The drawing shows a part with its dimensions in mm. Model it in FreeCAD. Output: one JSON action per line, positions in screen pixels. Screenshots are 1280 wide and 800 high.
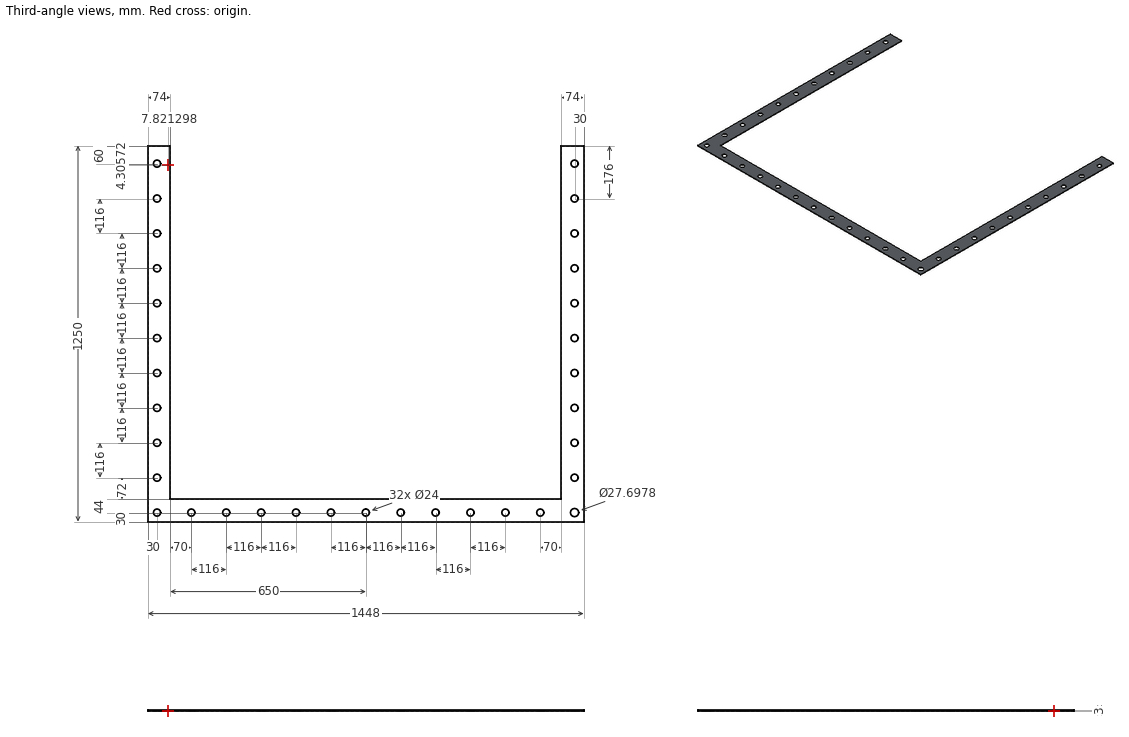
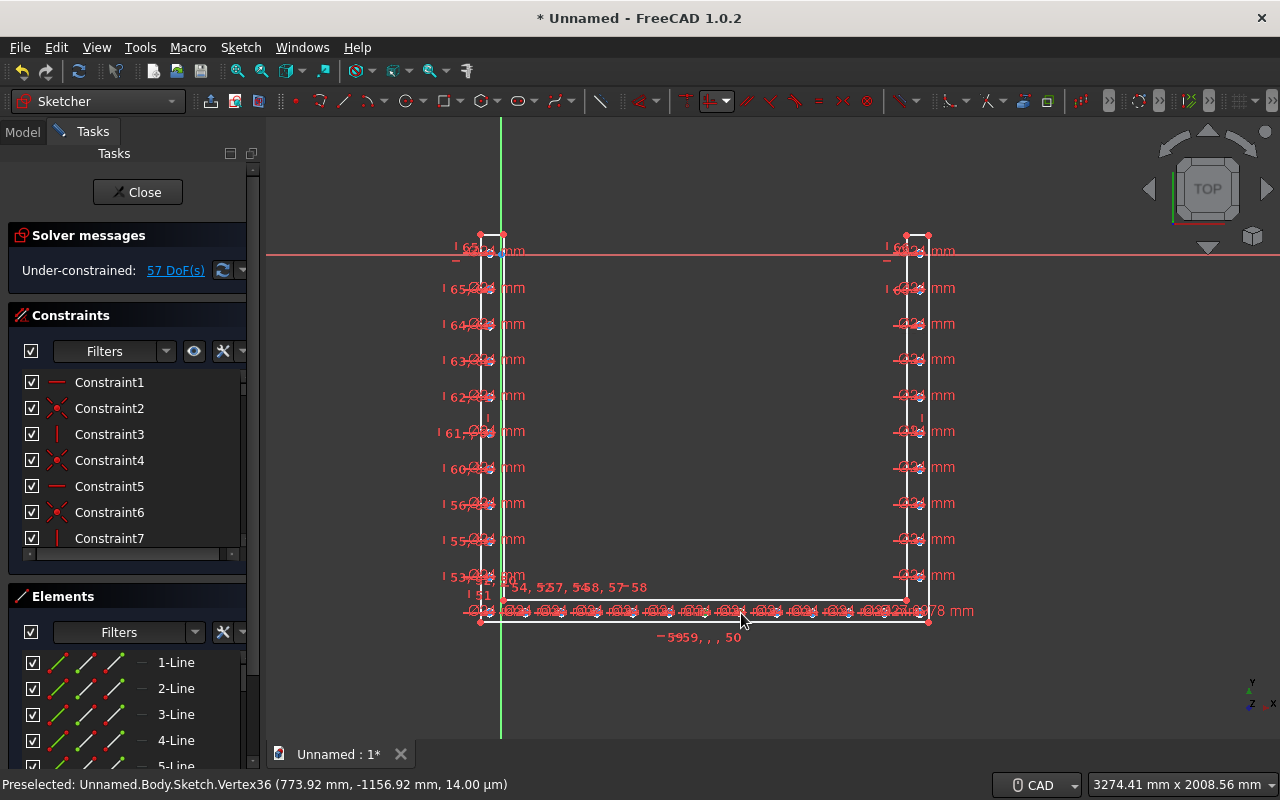
{"action": "left_click", "coordinate": [728, 102]}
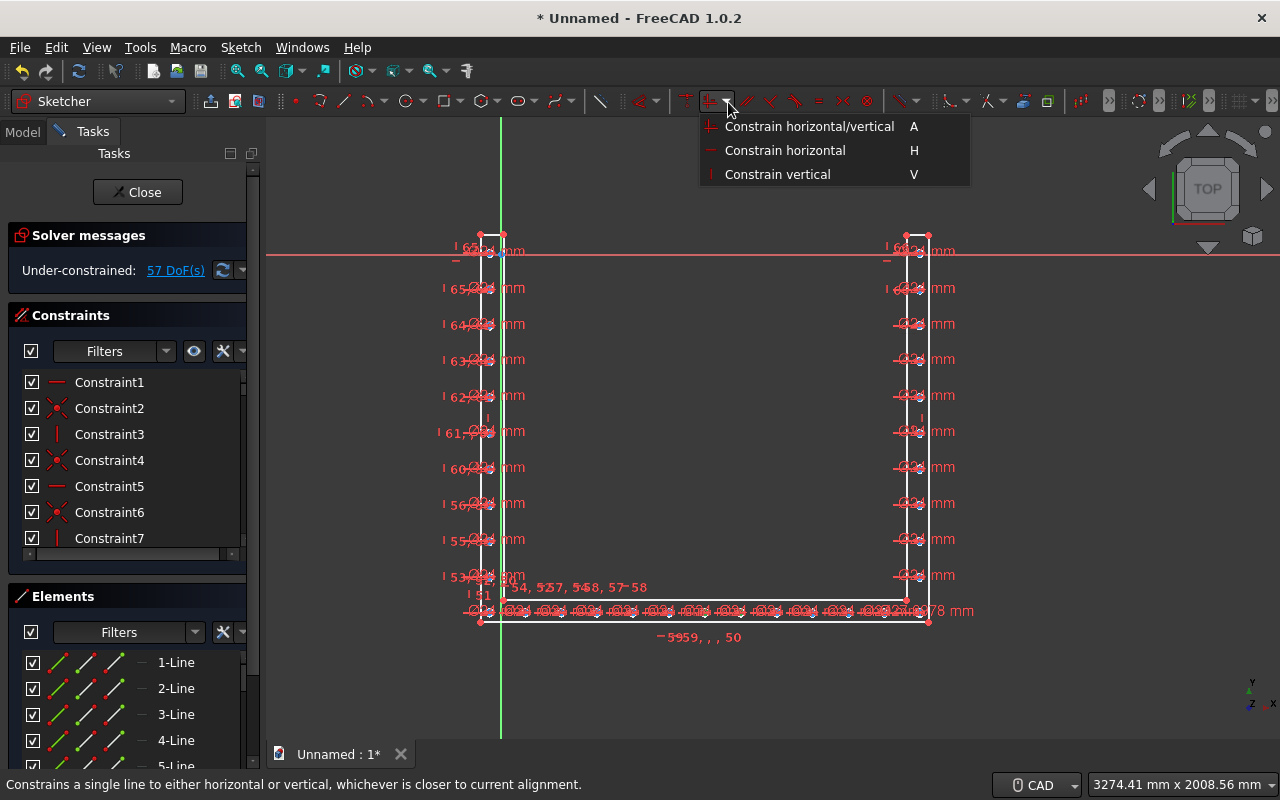
{"action": "left_click", "coordinate": [835, 150]}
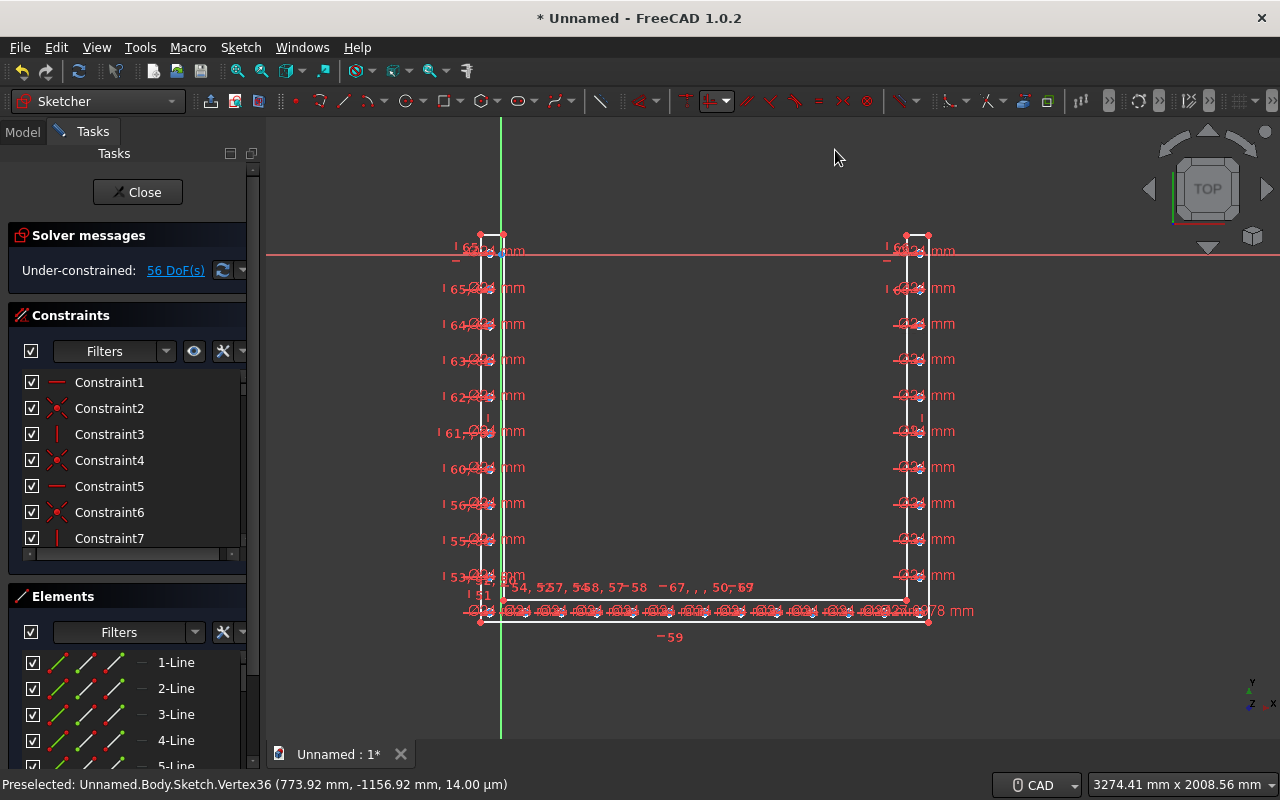
{"action": "left_click", "coordinate": [741, 613]}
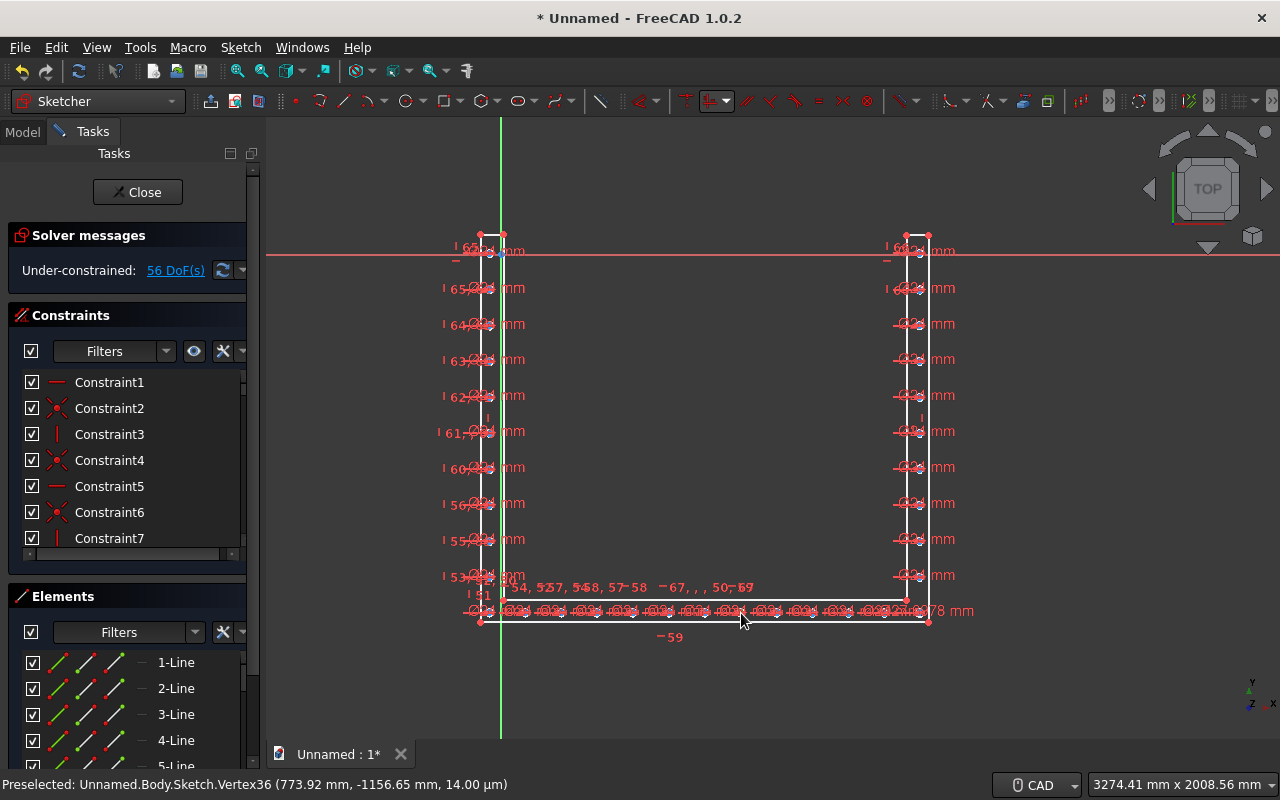
{"action": "left_click", "coordinate": [777, 613]}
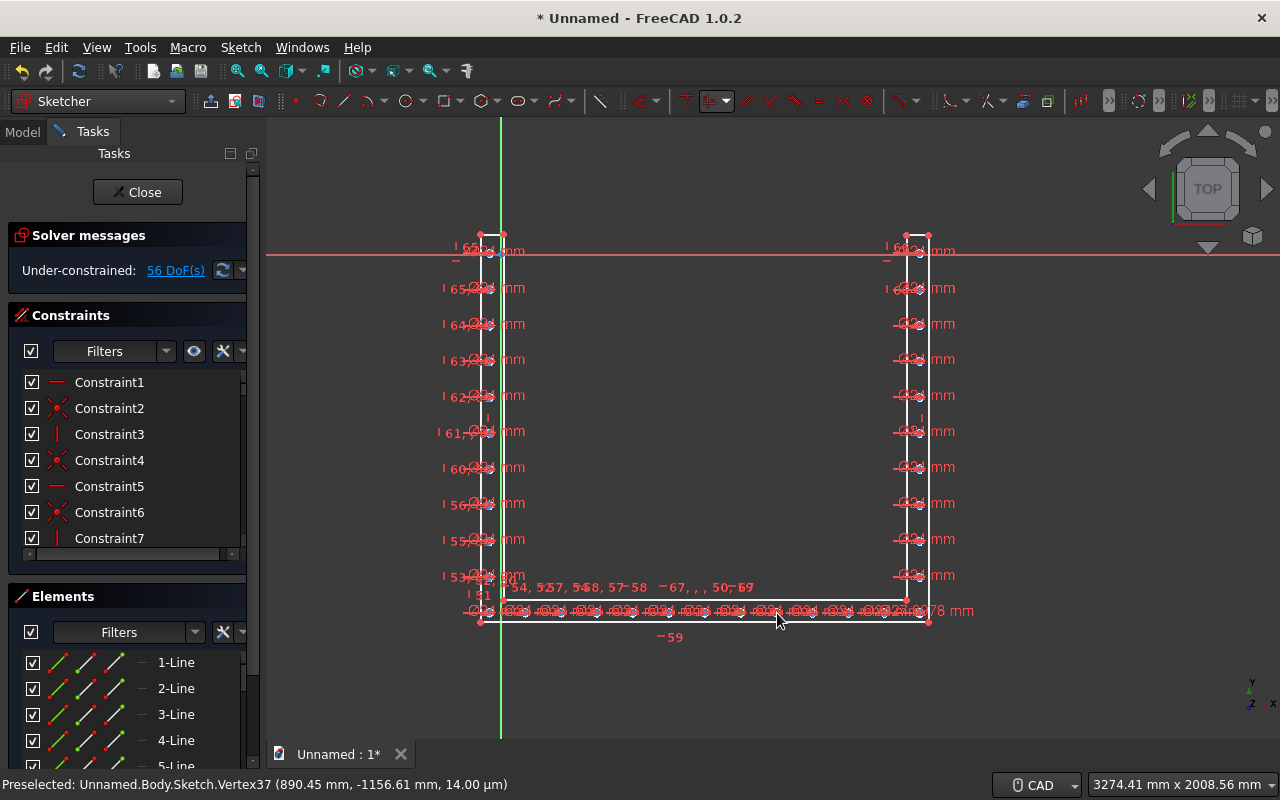
{"action": "left_click", "coordinate": [728, 102]}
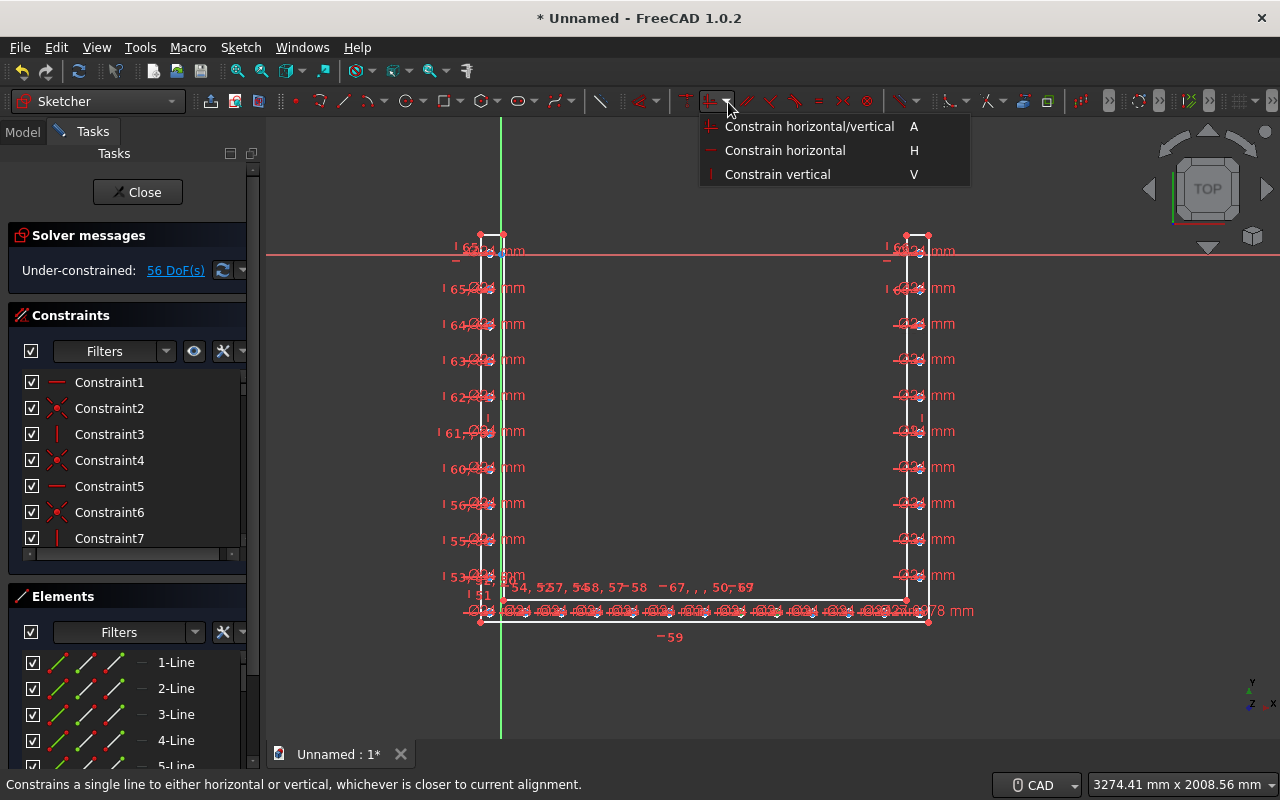
{"action": "left_click", "coordinate": [835, 150]}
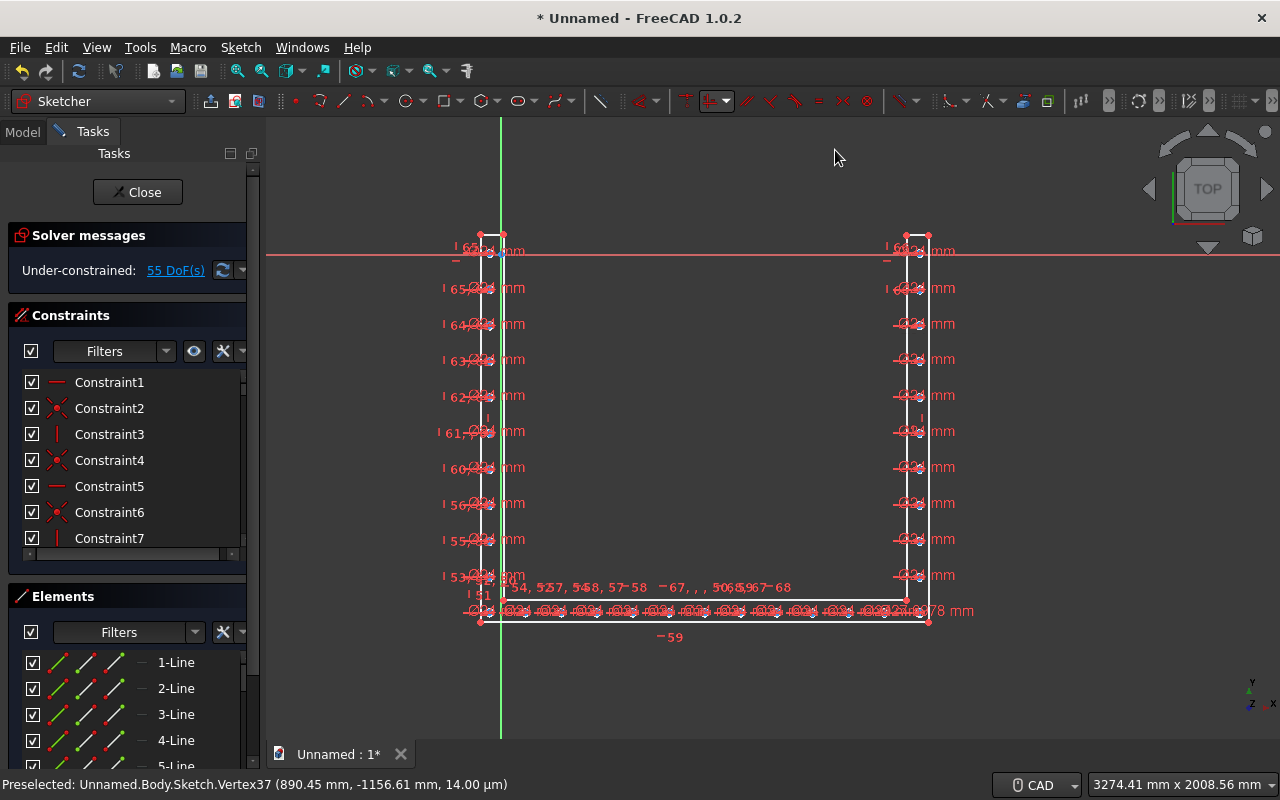
{"action": "left_click", "coordinate": [777, 613]}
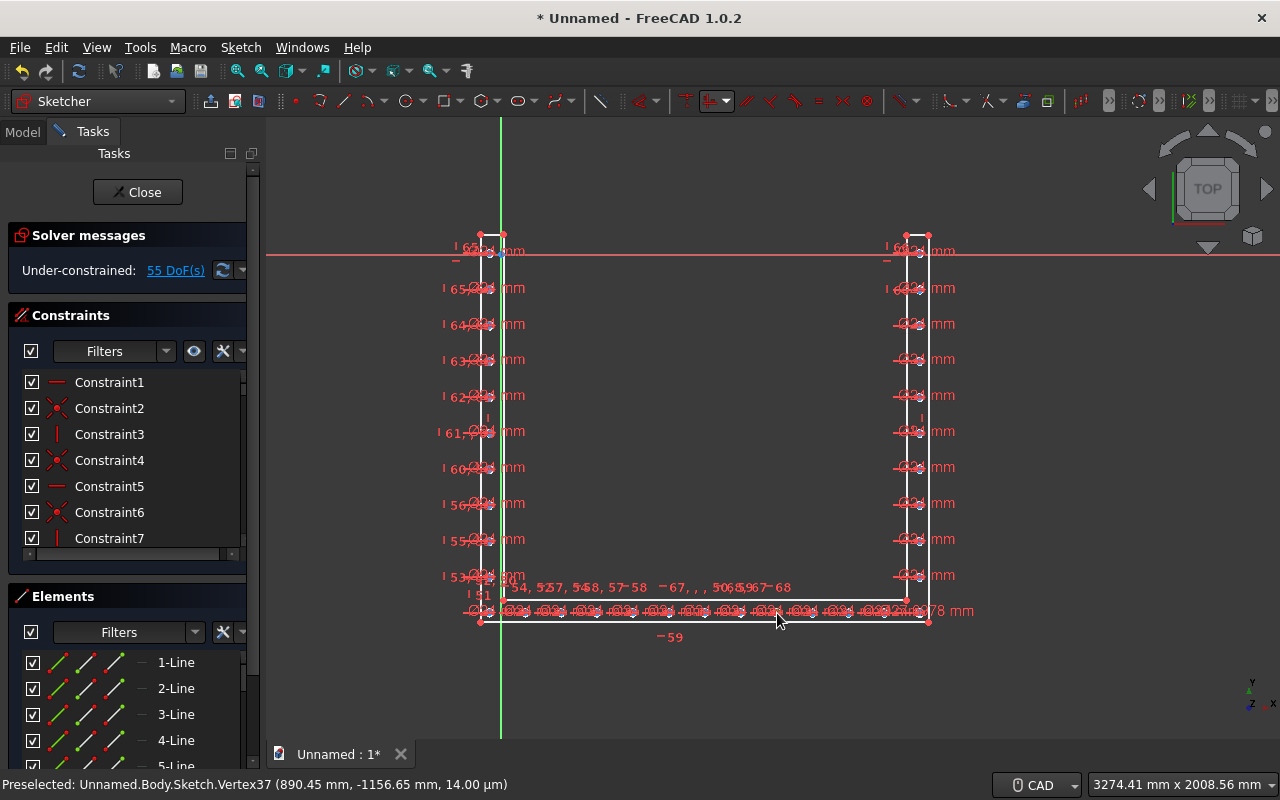
{"action": "left_click", "coordinate": [813, 613]}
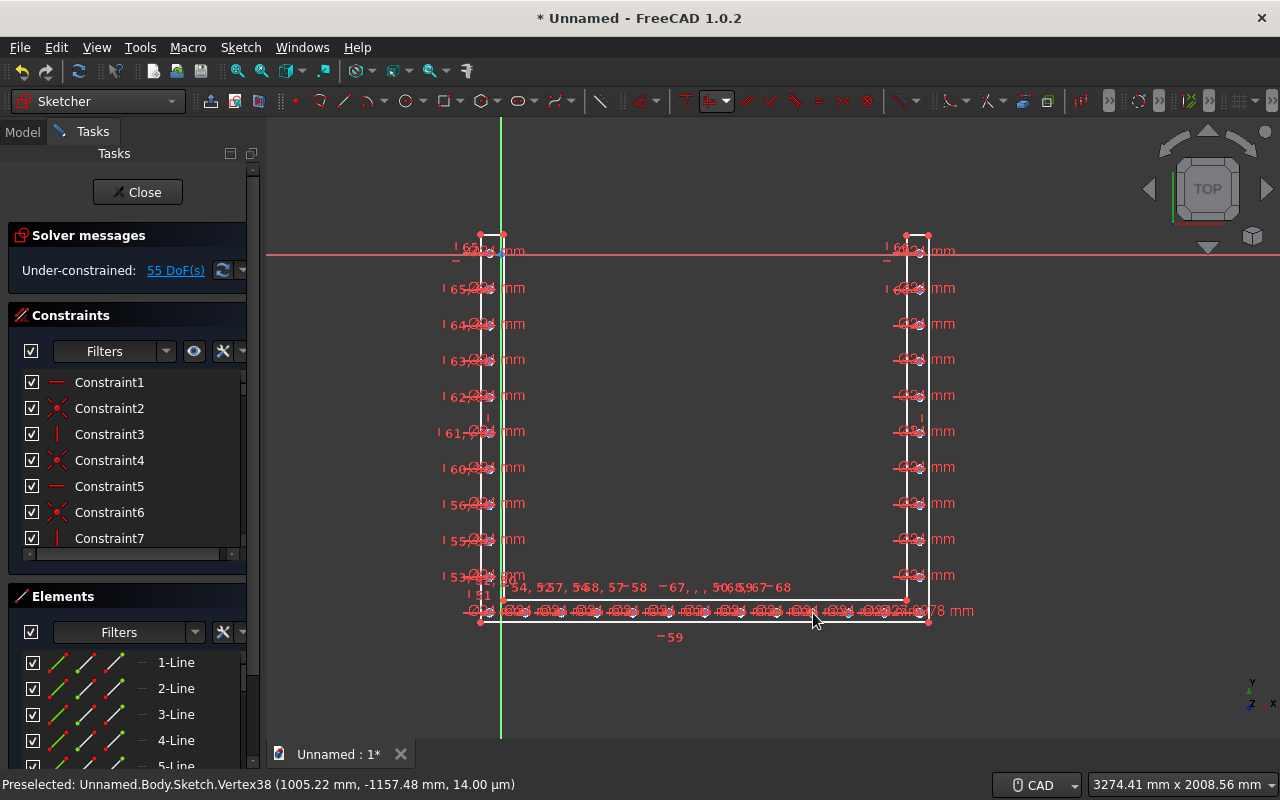
{"action": "left_click", "coordinate": [728, 102]}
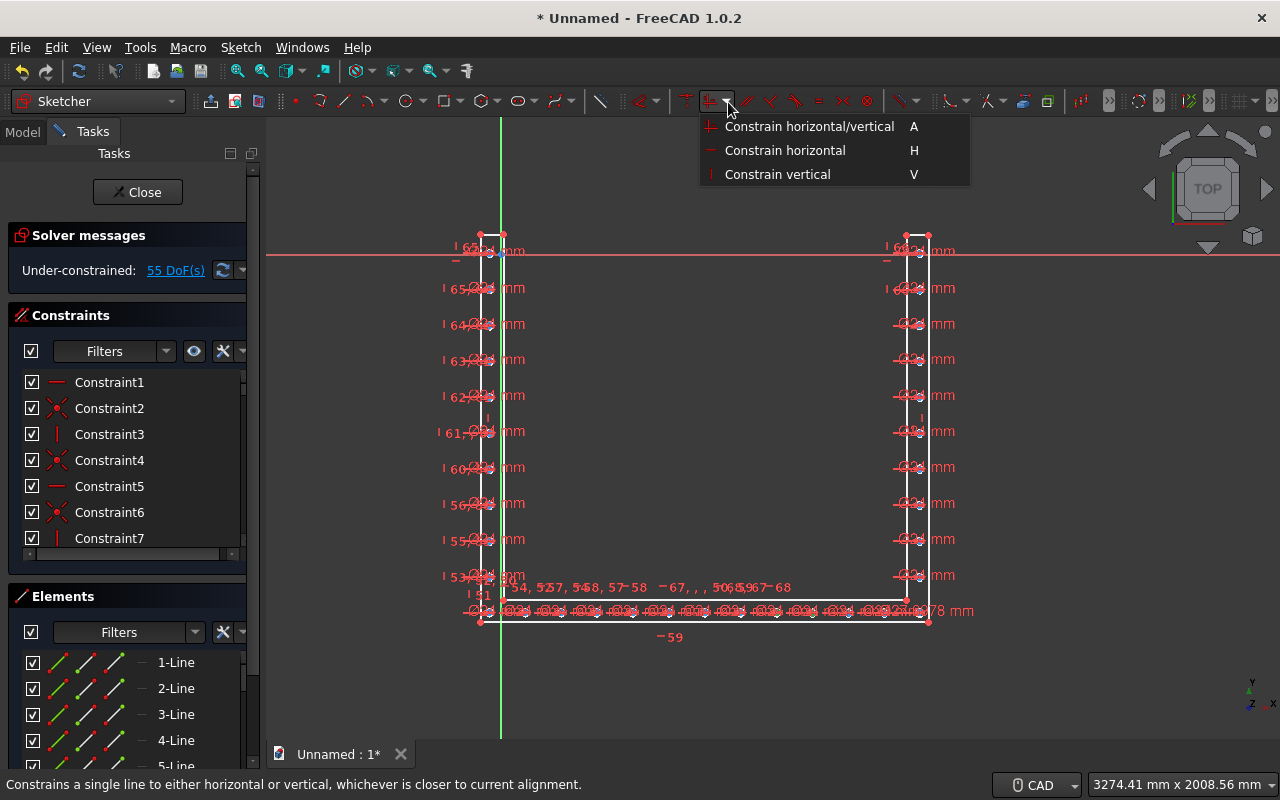
{"action": "left_click", "coordinate": [835, 150]}